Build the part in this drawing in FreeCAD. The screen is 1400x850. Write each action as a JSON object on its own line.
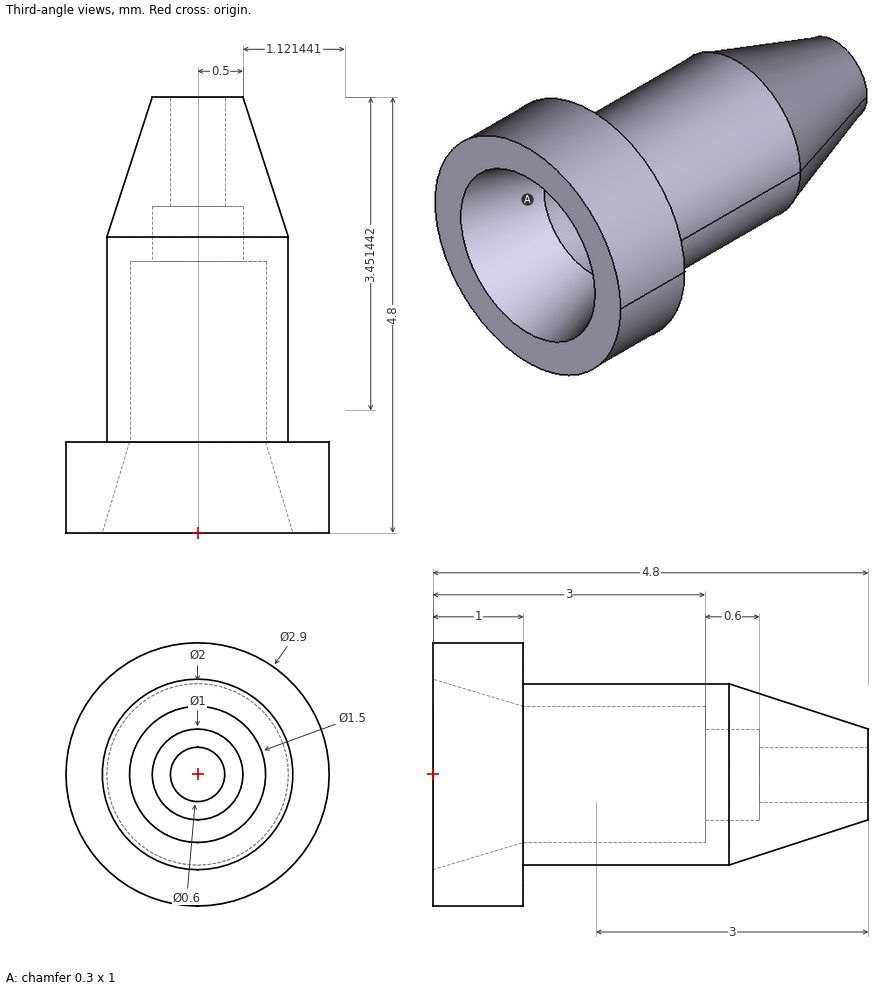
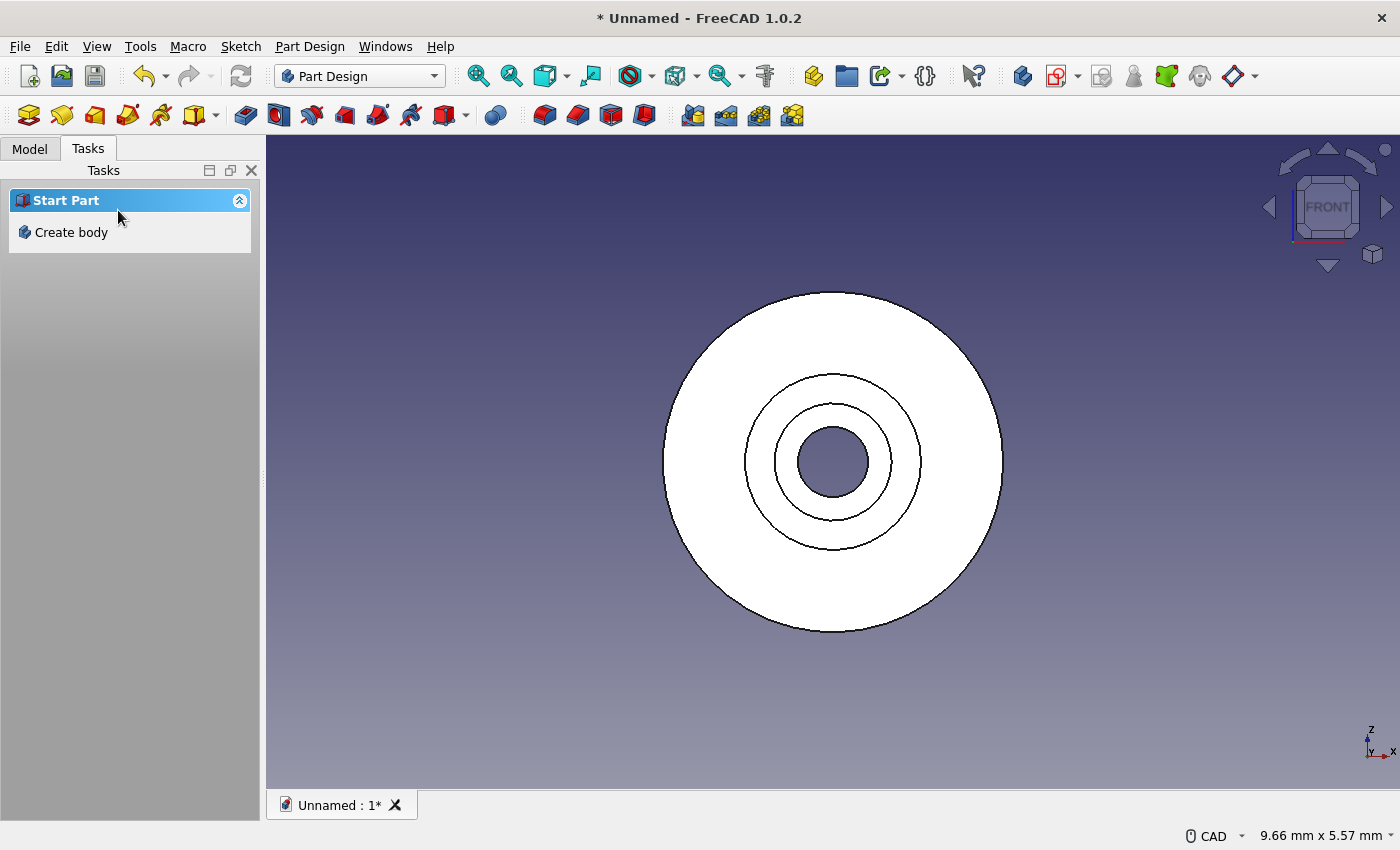
{"action": "left_click", "coordinate": [762, 409]}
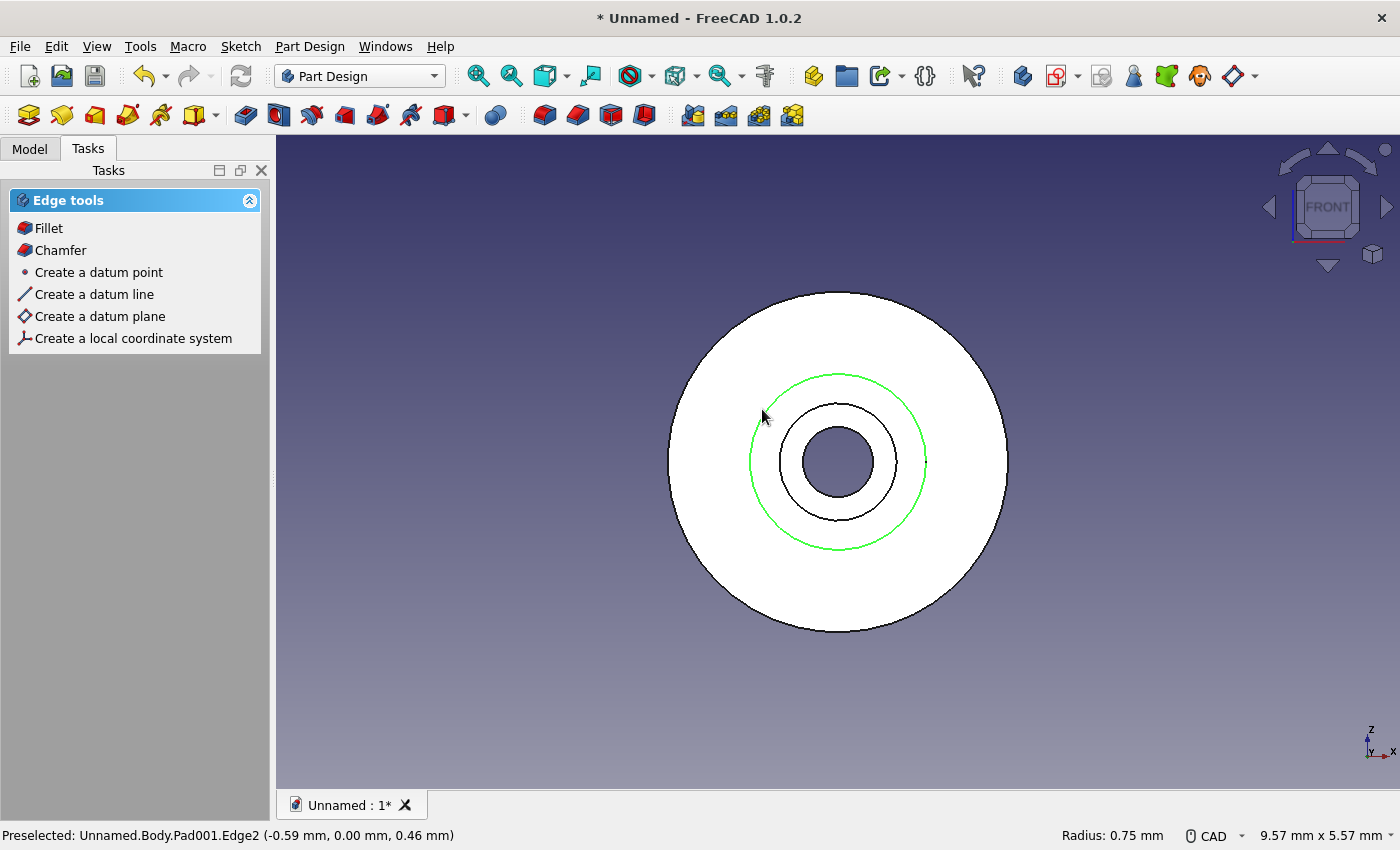
{"action": "left_click", "coordinate": [578, 116]}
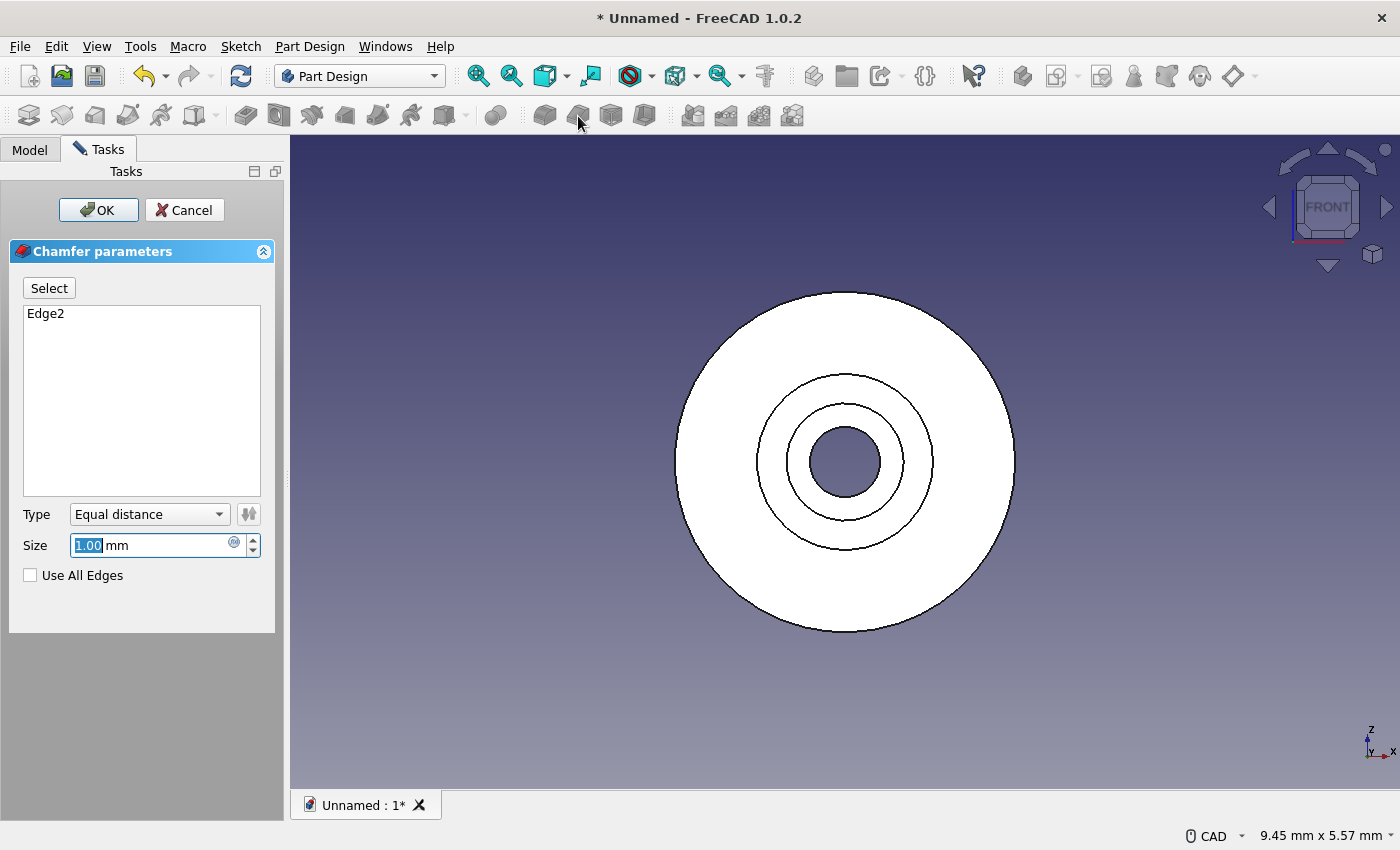
{"action": "type", "text": "0.3"}
{"action": "key", "text": "Tab"}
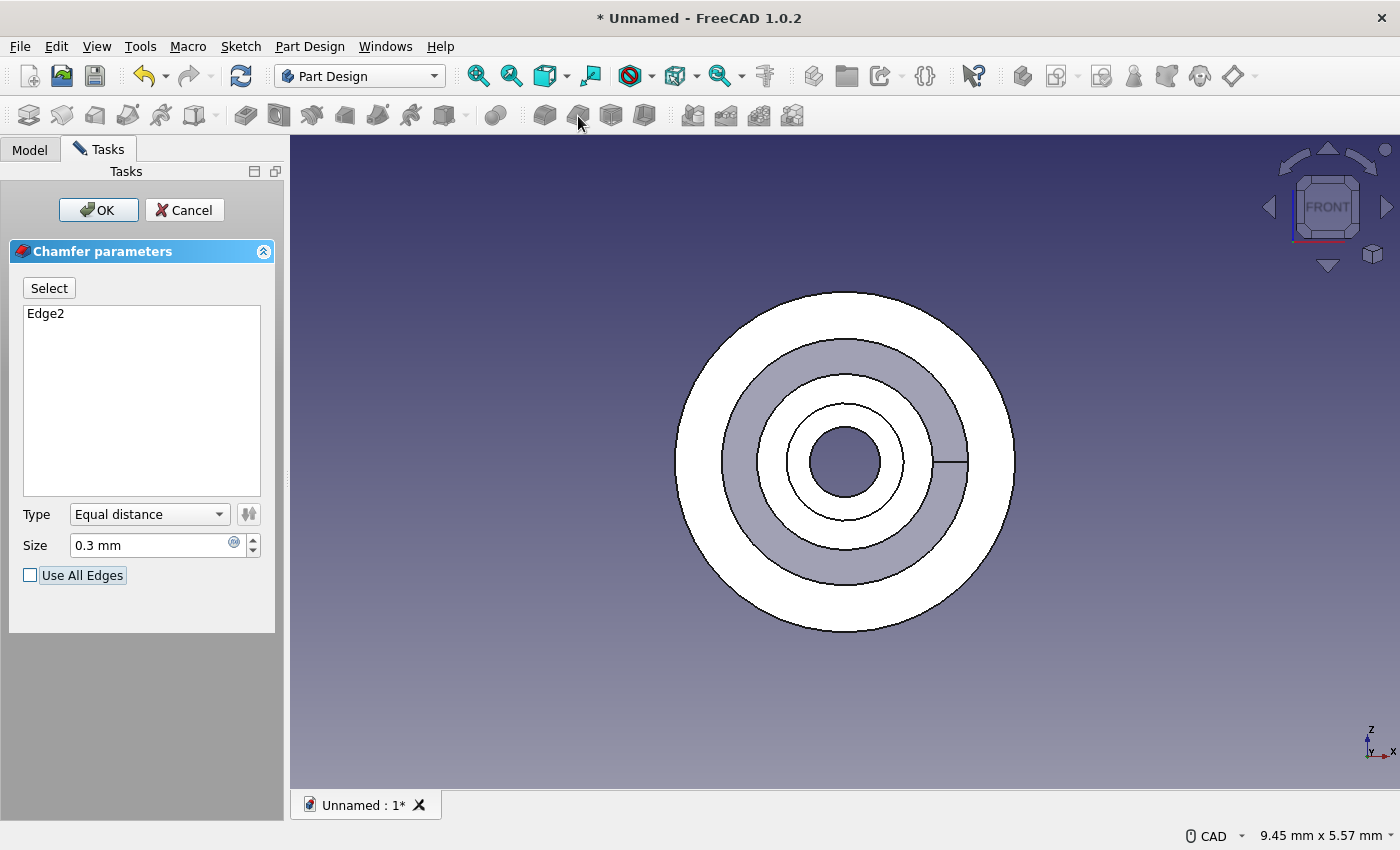
{"action": "left_click", "coordinate": [150, 514]}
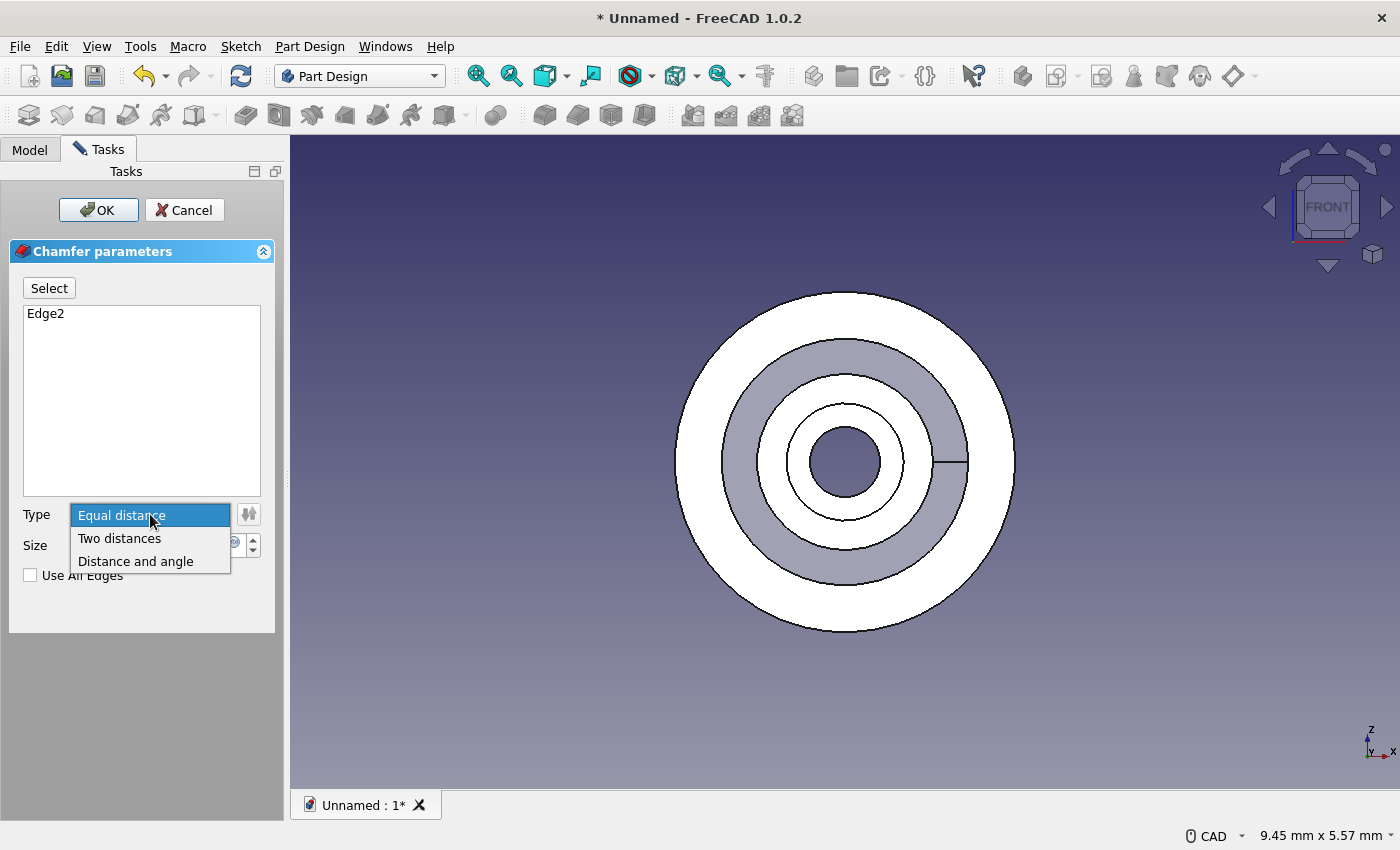
{"action": "left_click", "coordinate": [148, 538]}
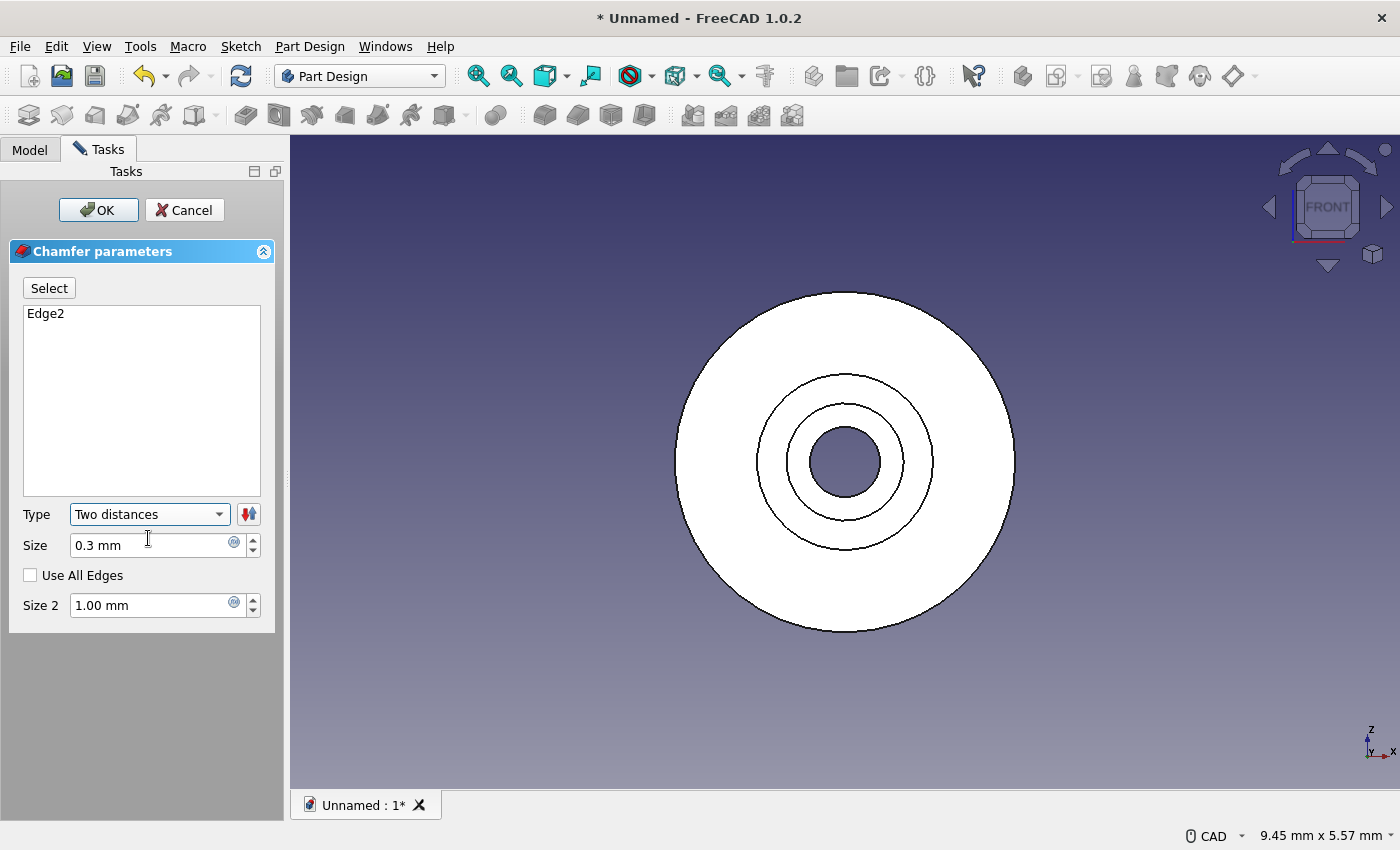
{"action": "triple_click", "coordinate": [158, 606]}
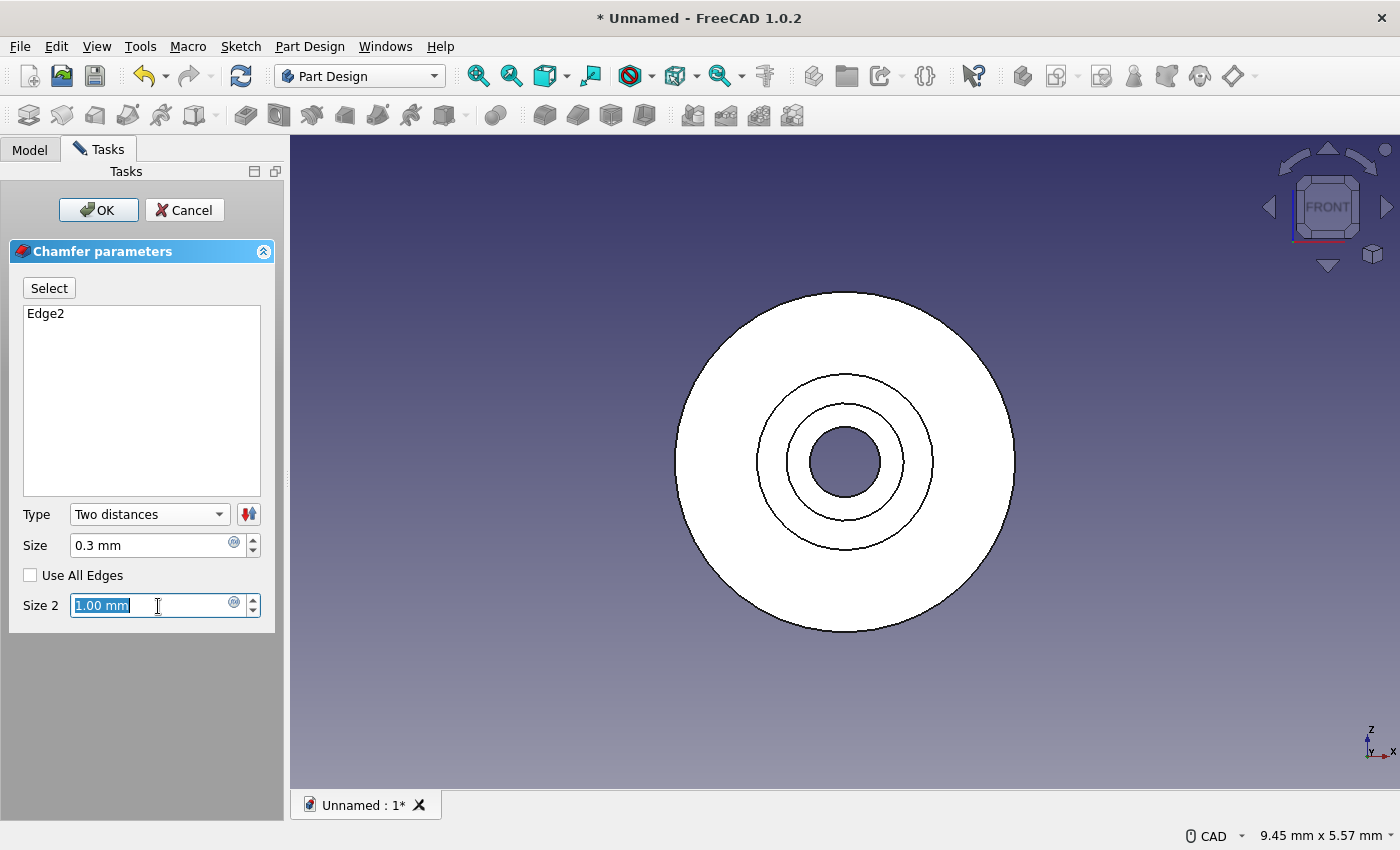
{"action": "type", "text": "1"}
{"action": "key", "text": "Tab"}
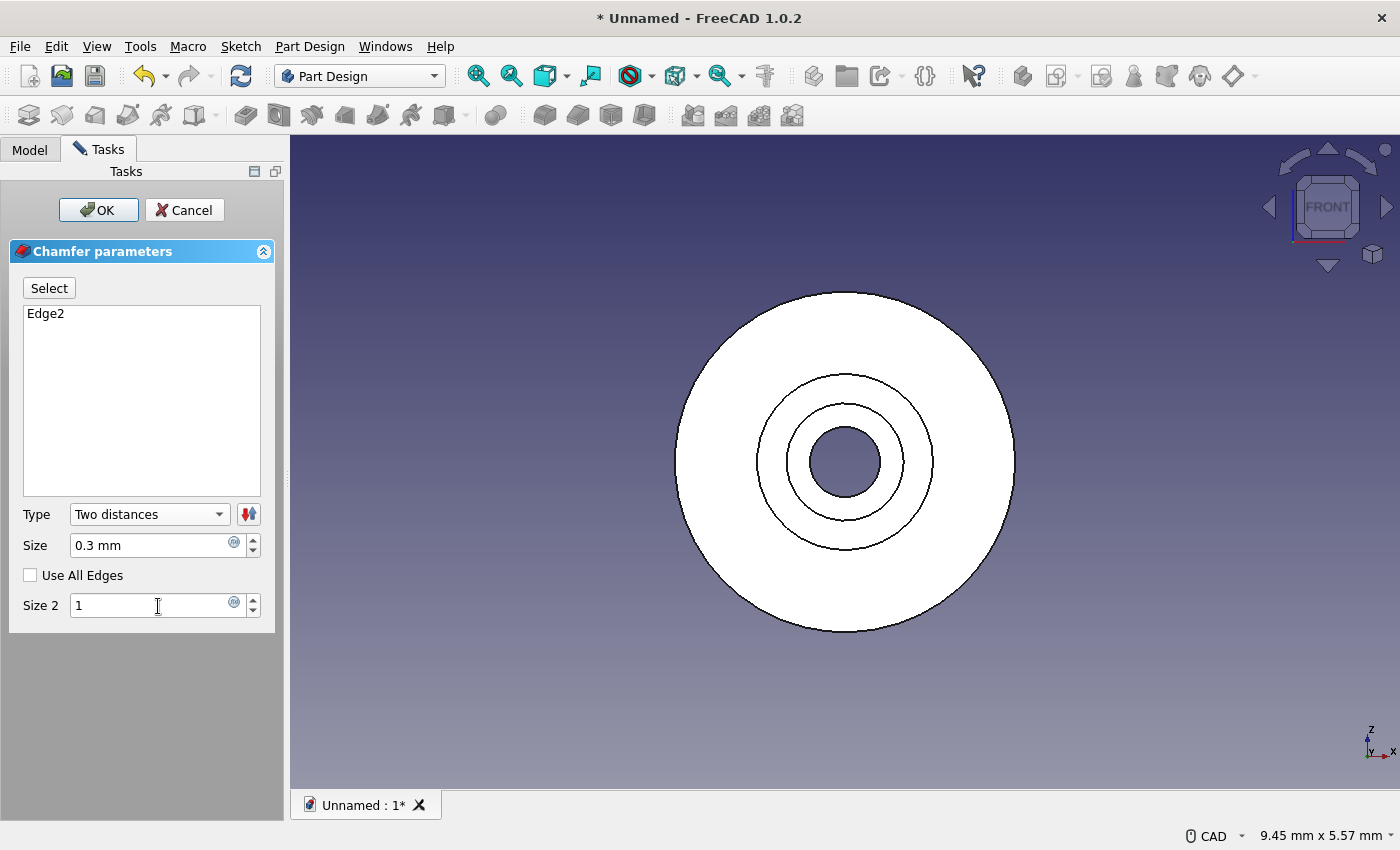
{"action": "left_click", "coordinate": [249, 514]}